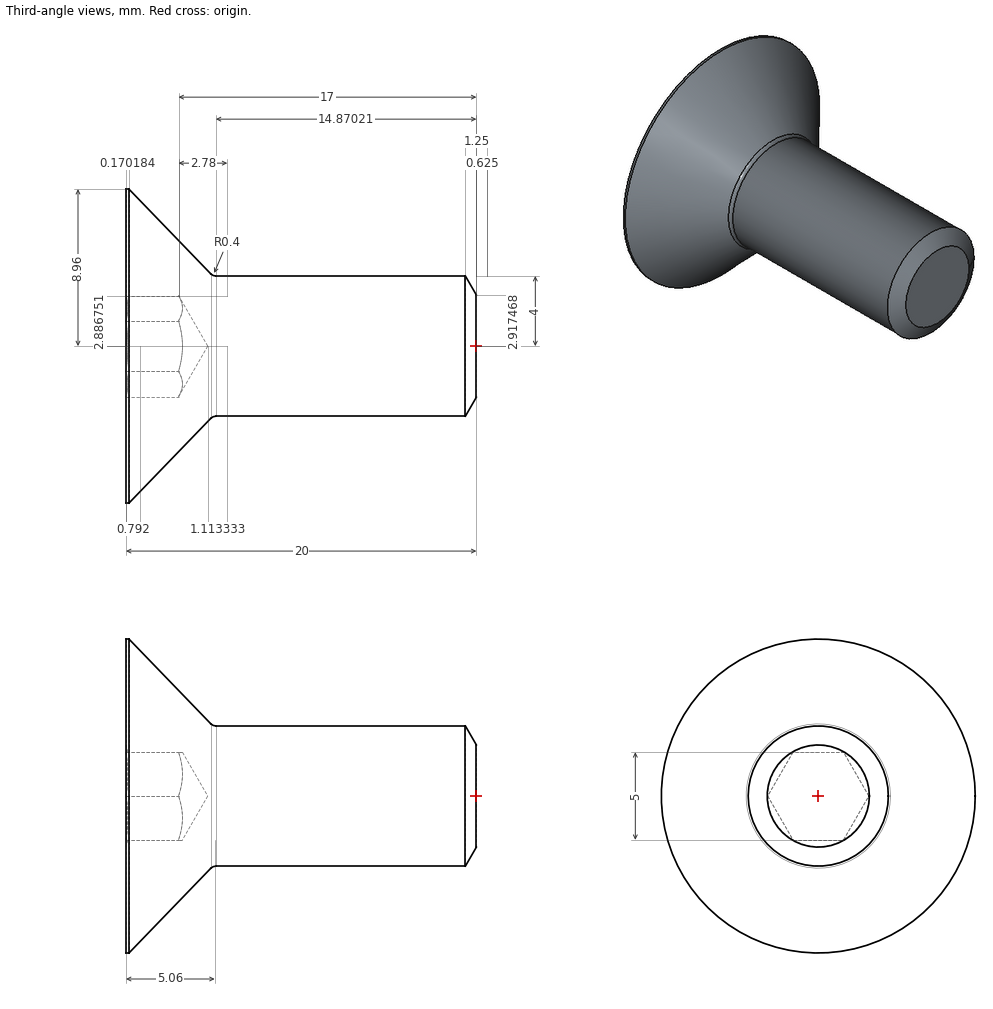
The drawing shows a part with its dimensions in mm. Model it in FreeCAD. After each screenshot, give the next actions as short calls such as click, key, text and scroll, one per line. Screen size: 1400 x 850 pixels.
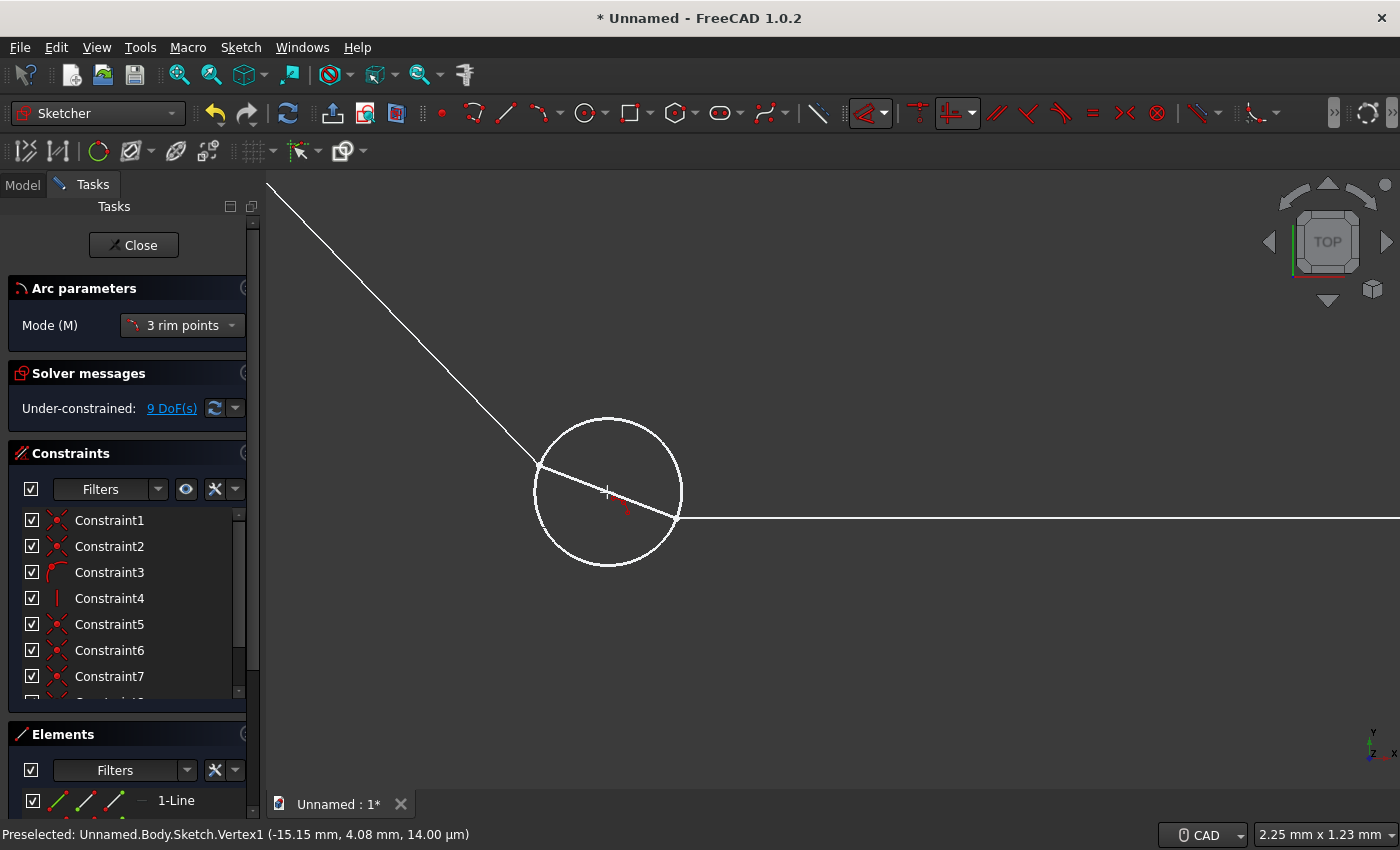
click(601, 491)
key(Escape)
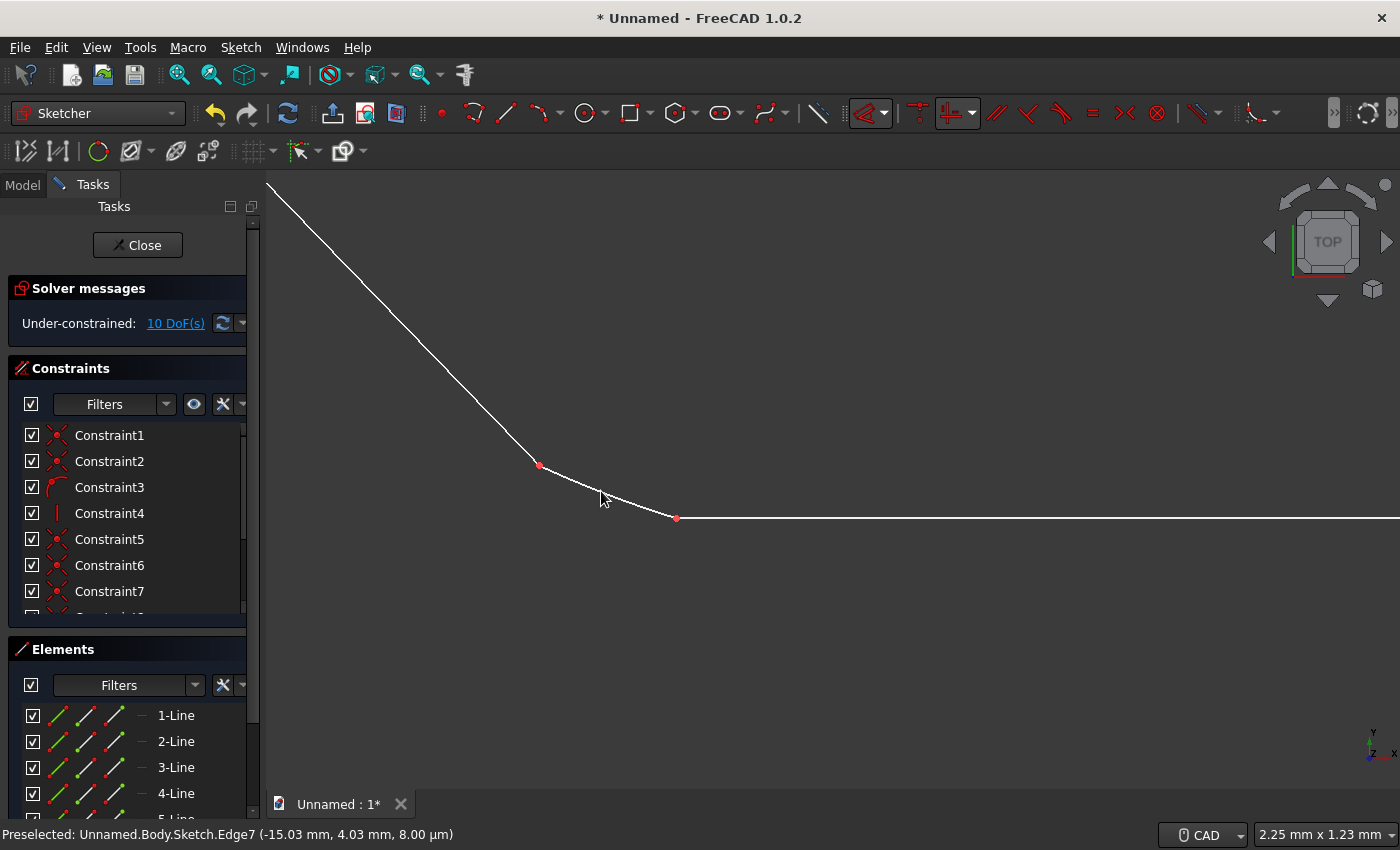
scroll(611, 493, down, 14)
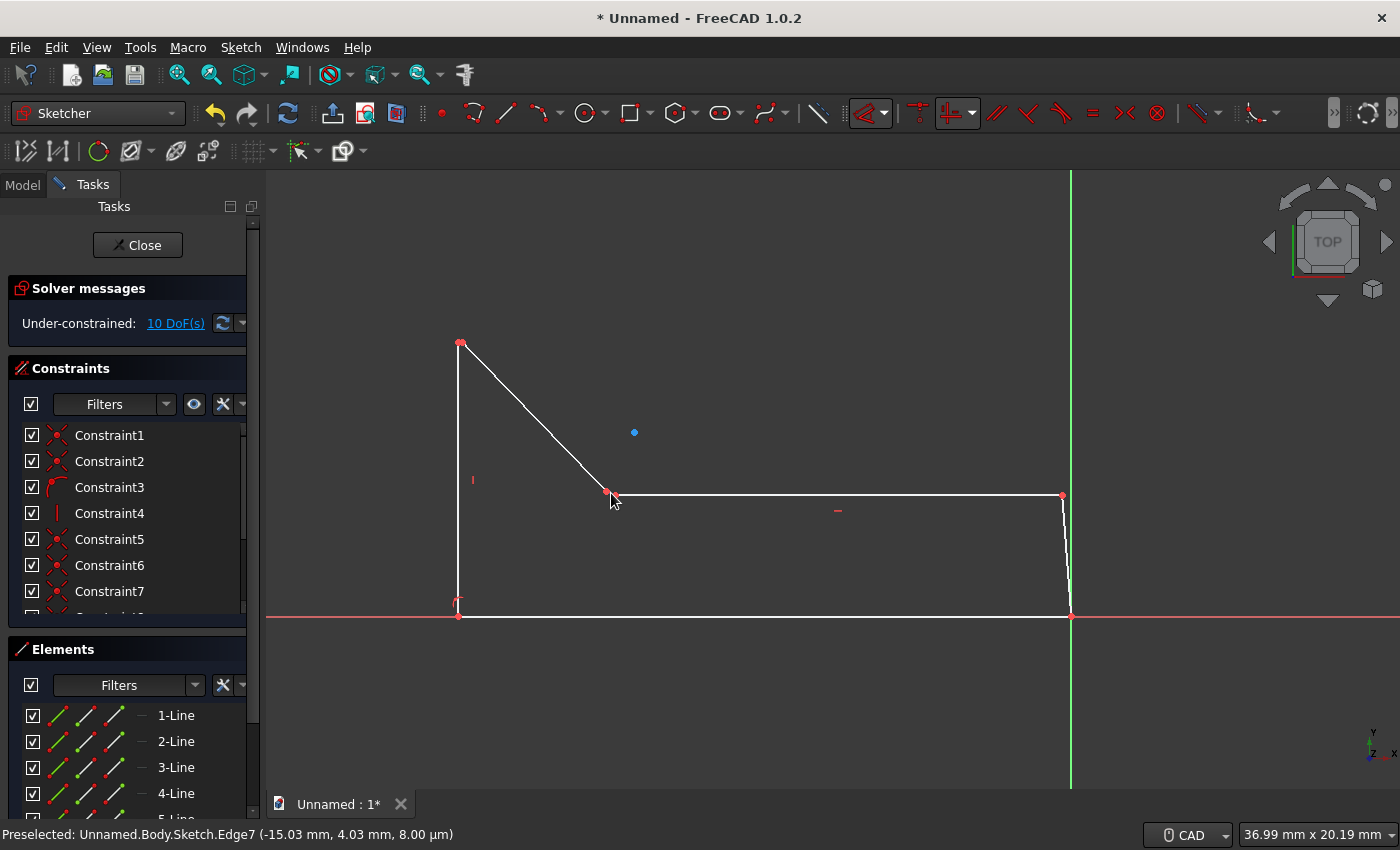
click(564, 447)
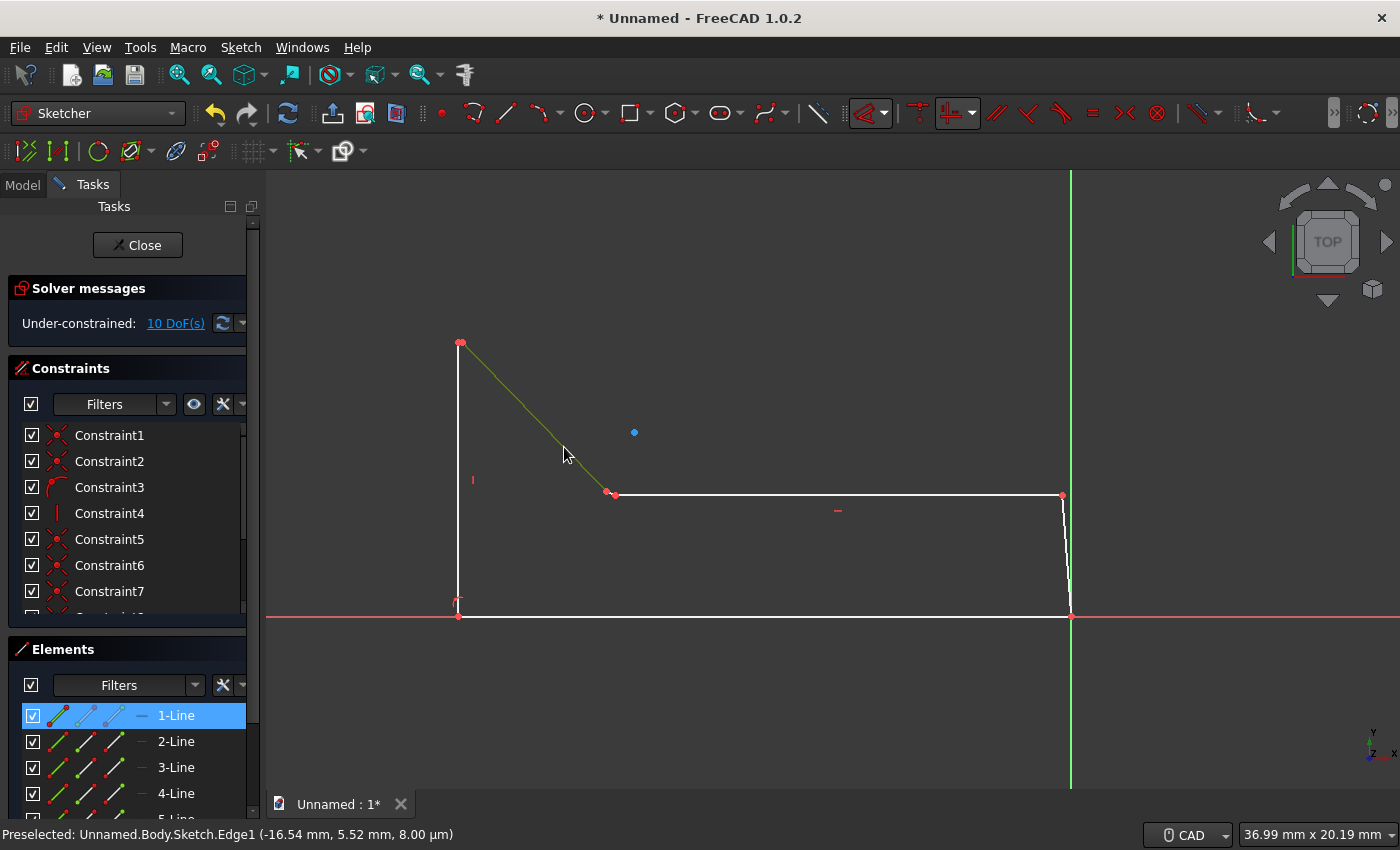
scroll(611, 494, up, 6)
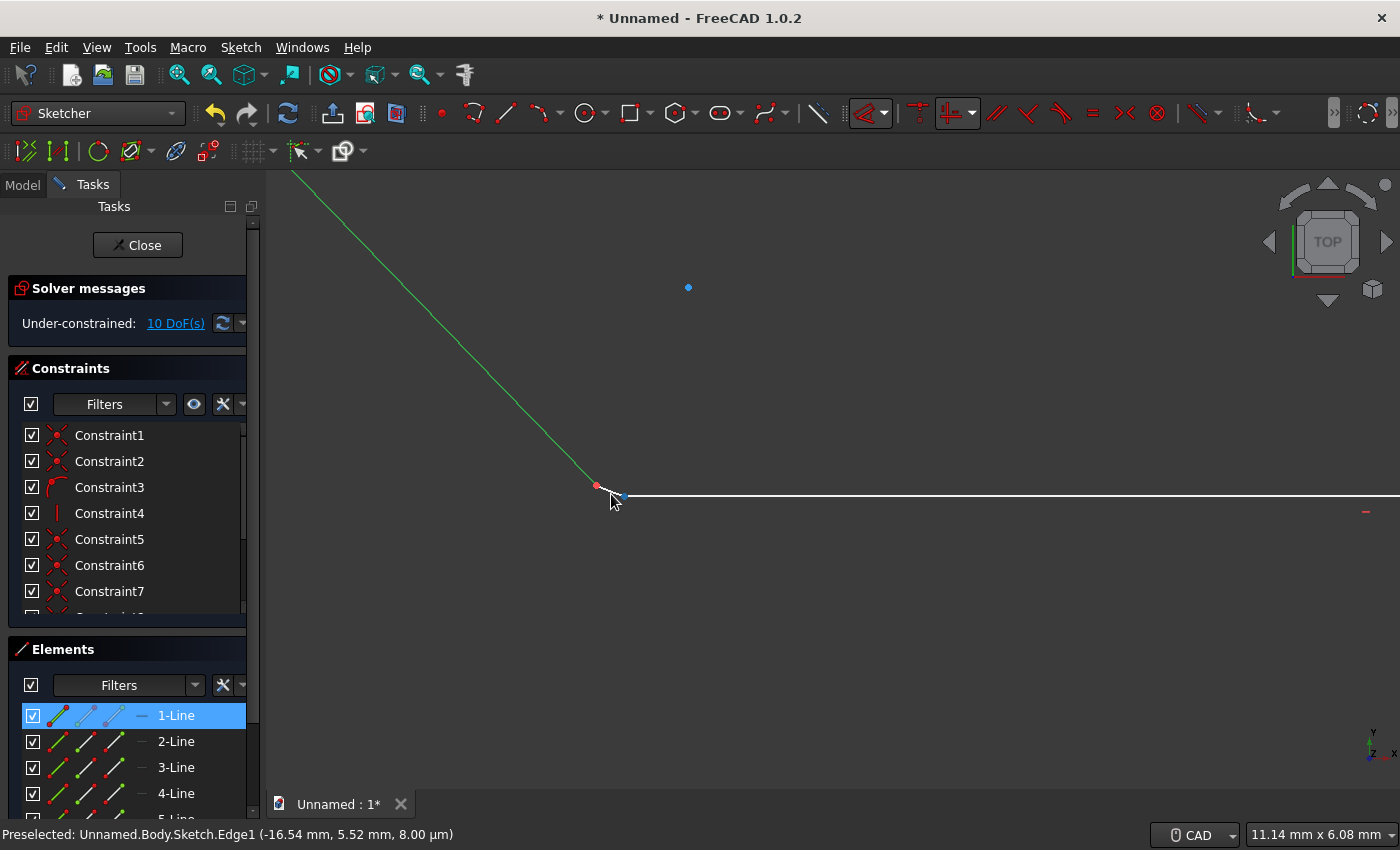
click(610, 491)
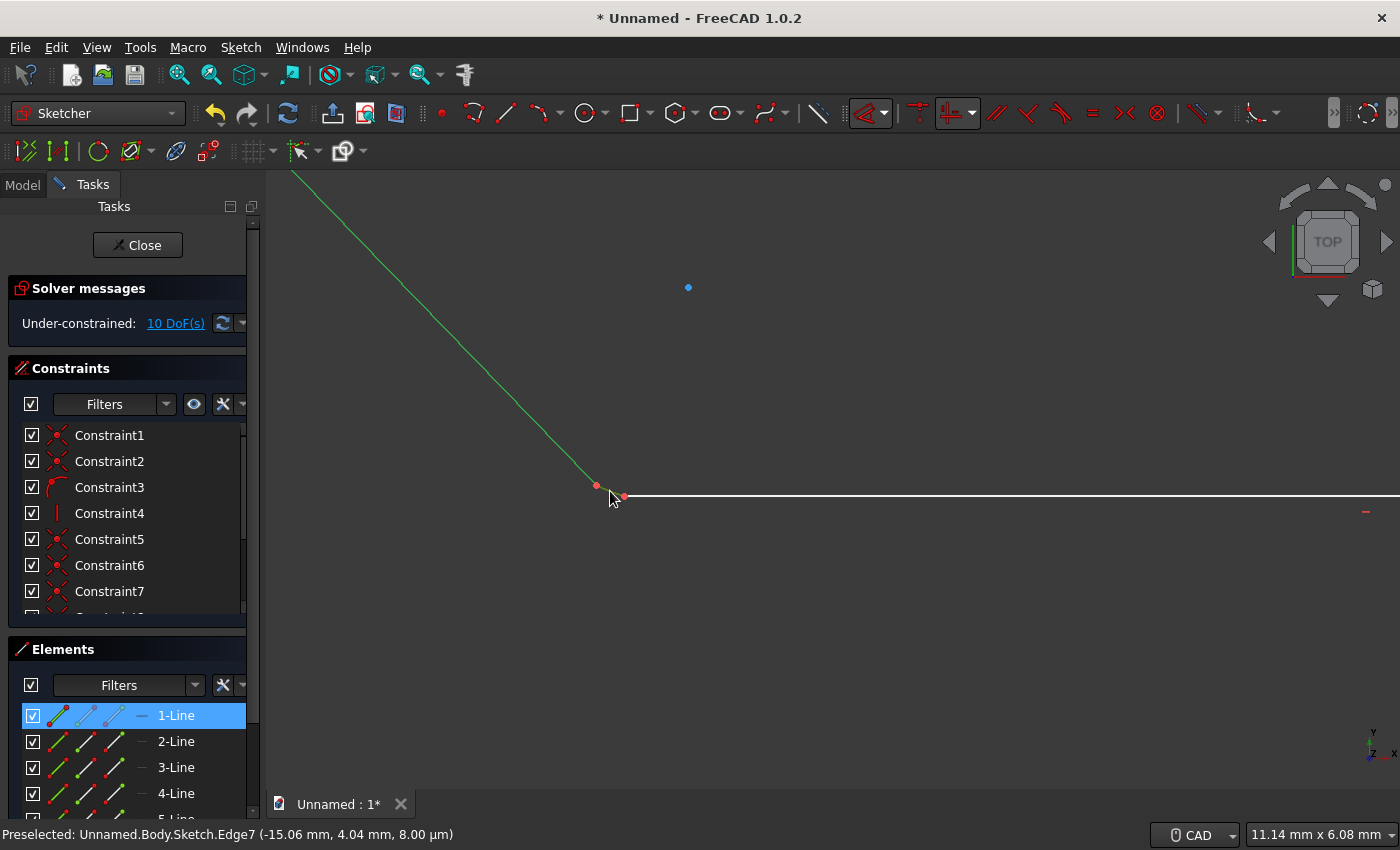
click(1062, 114)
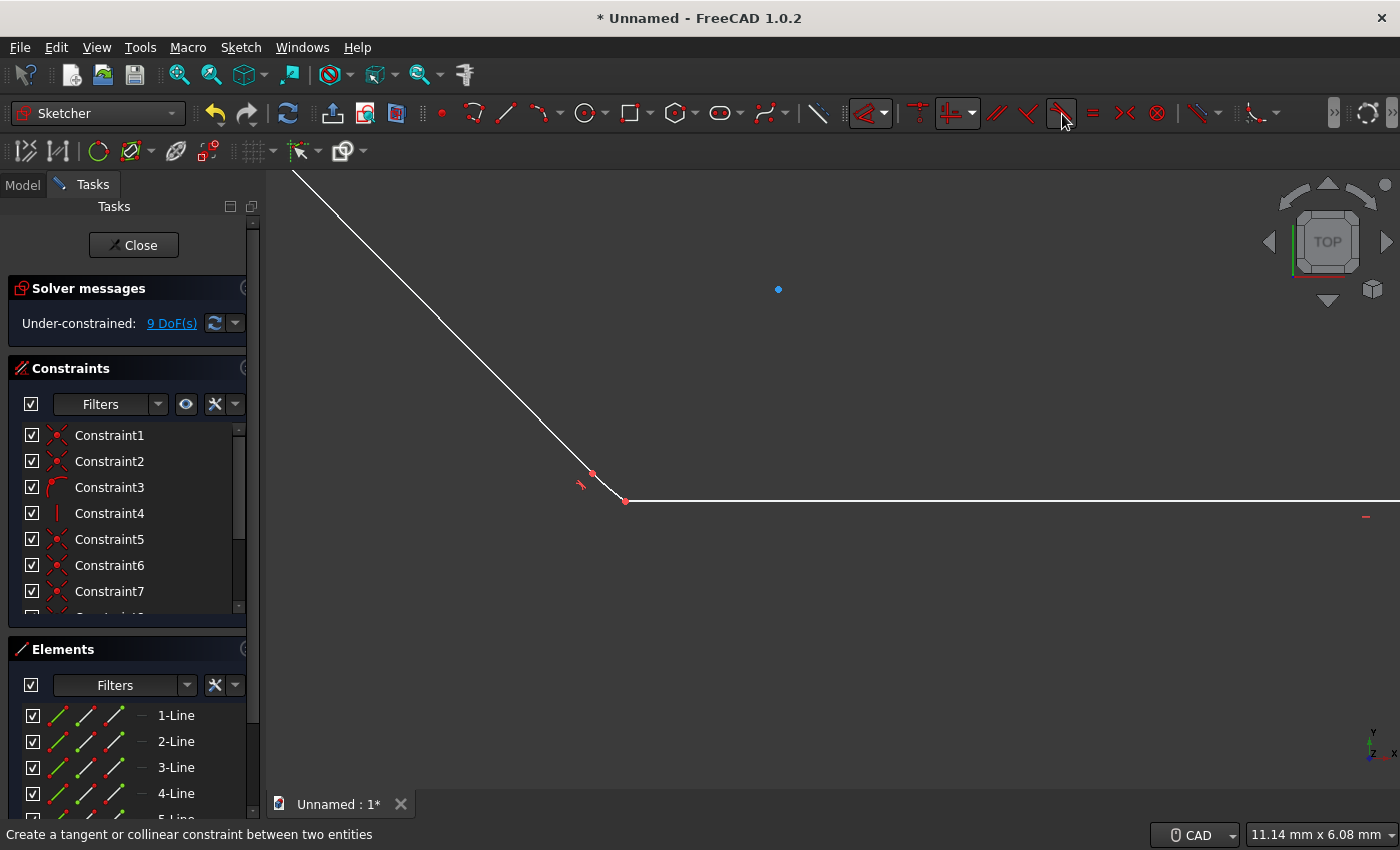
click(1070, 501)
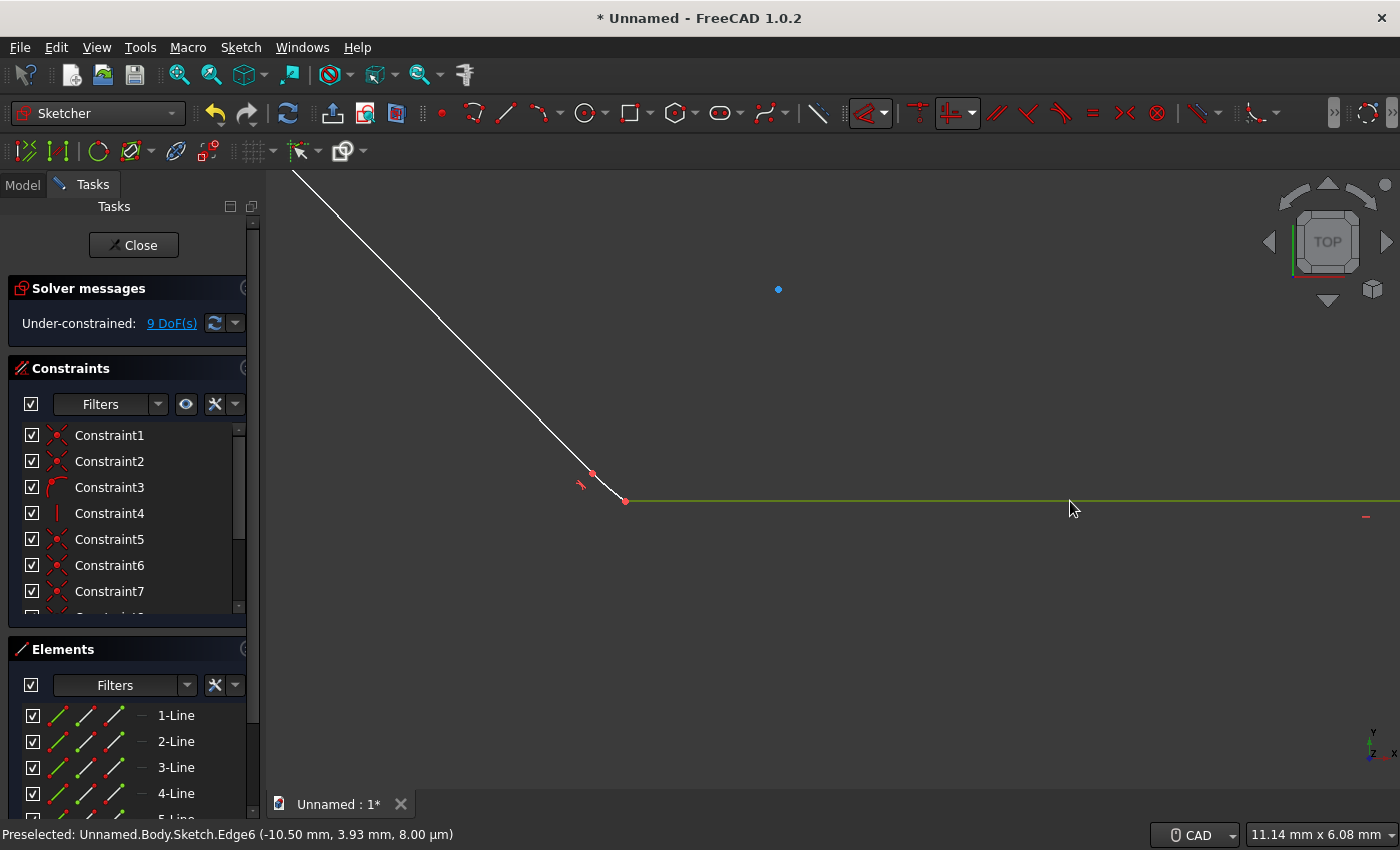
click(602, 482)